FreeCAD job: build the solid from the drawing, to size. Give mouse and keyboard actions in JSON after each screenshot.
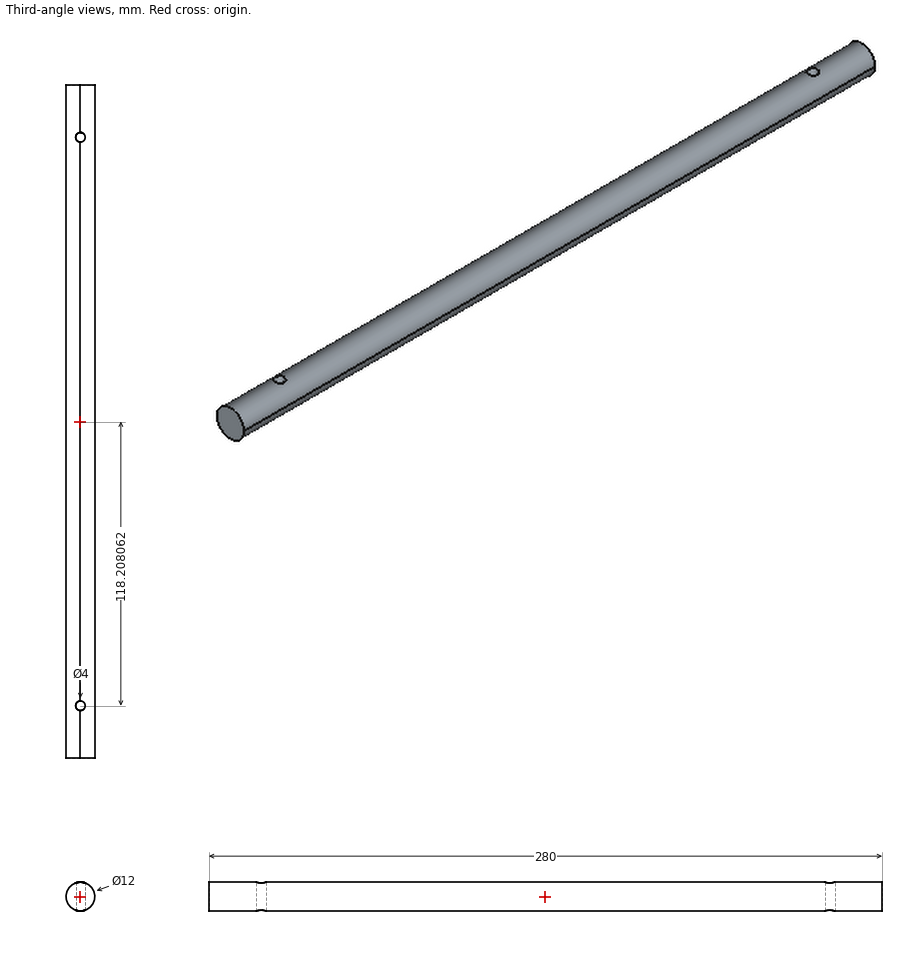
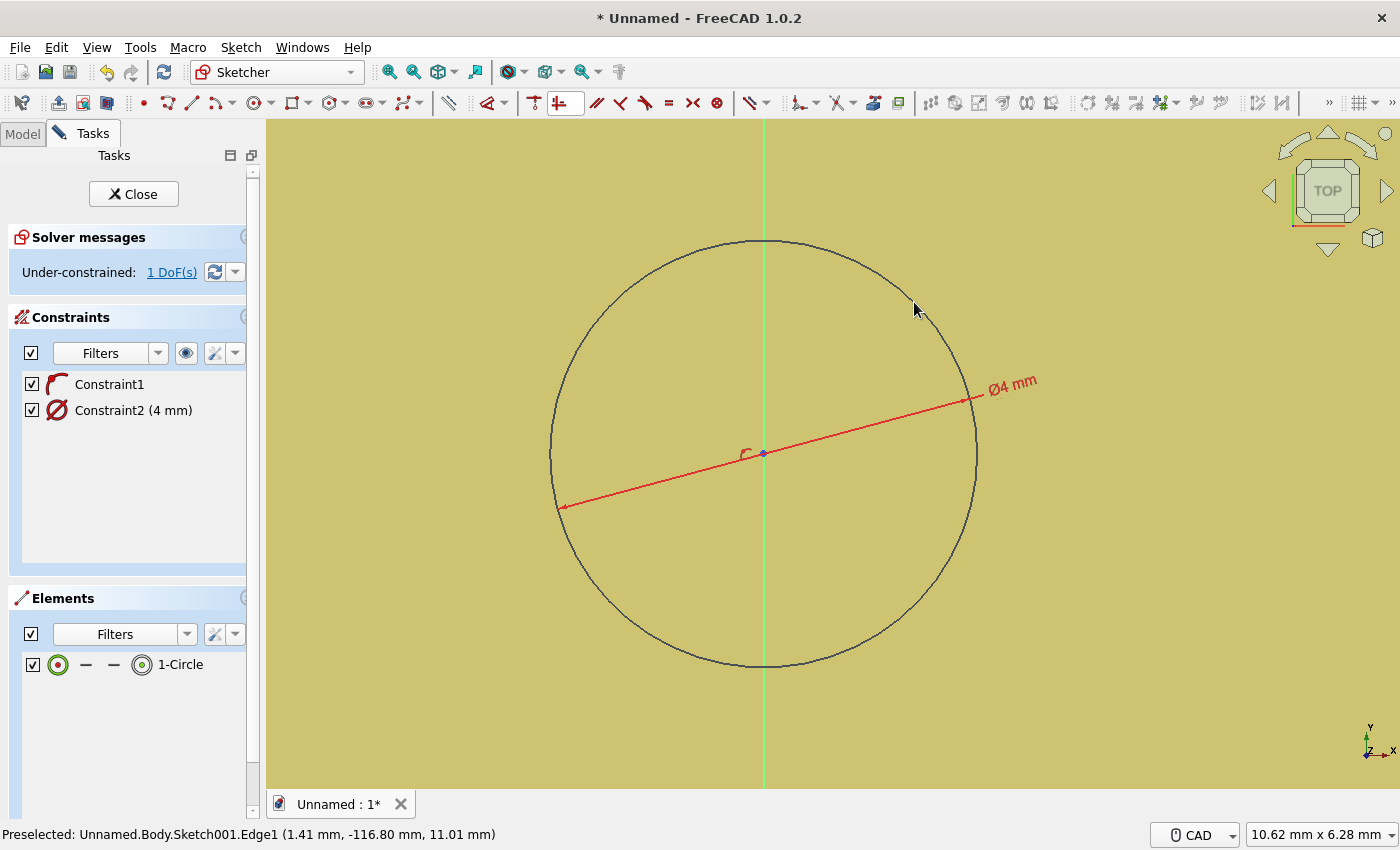
{"action": "left_click", "coordinate": [764, 454]}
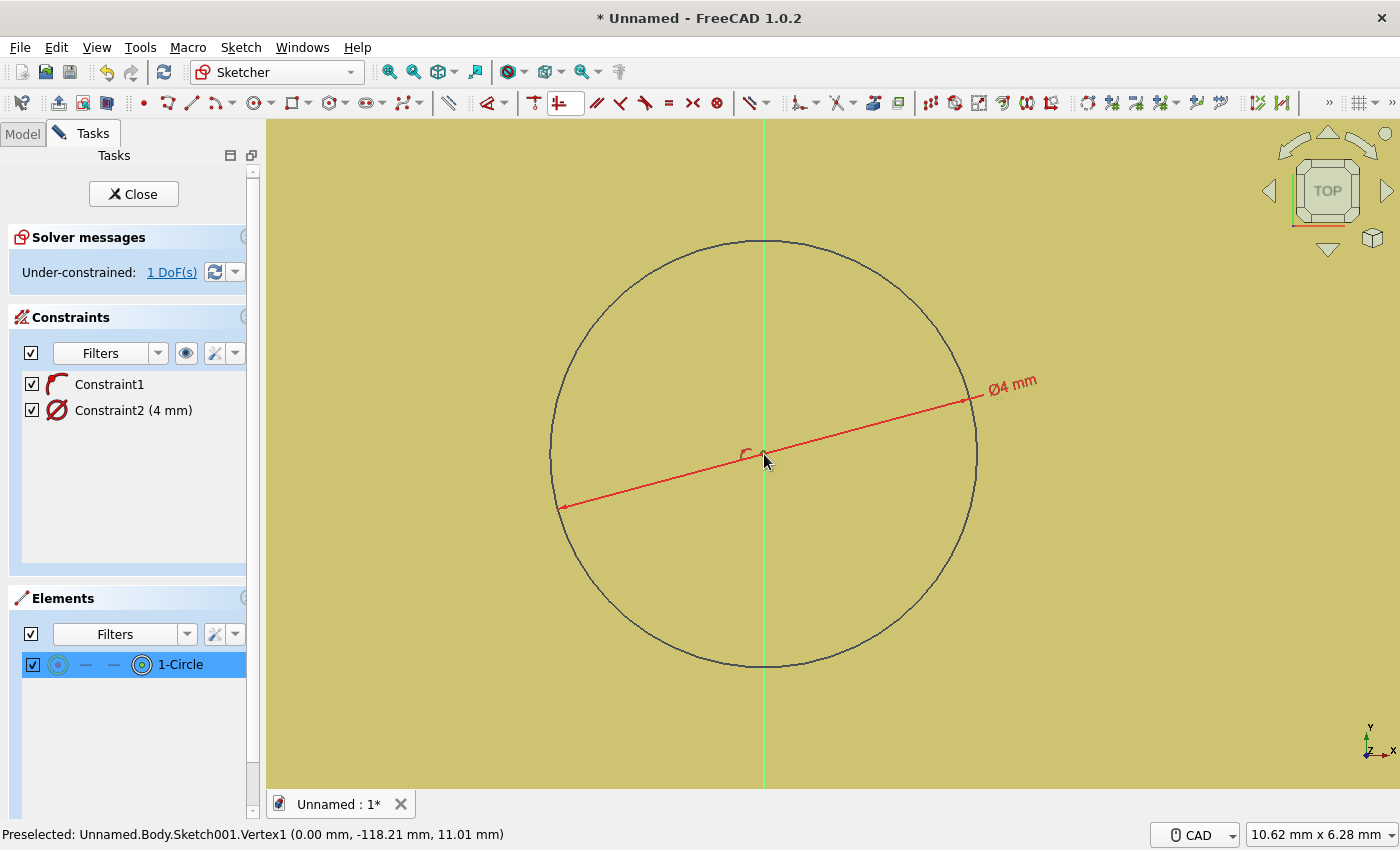
{"action": "left_click", "coordinate": [506, 104]}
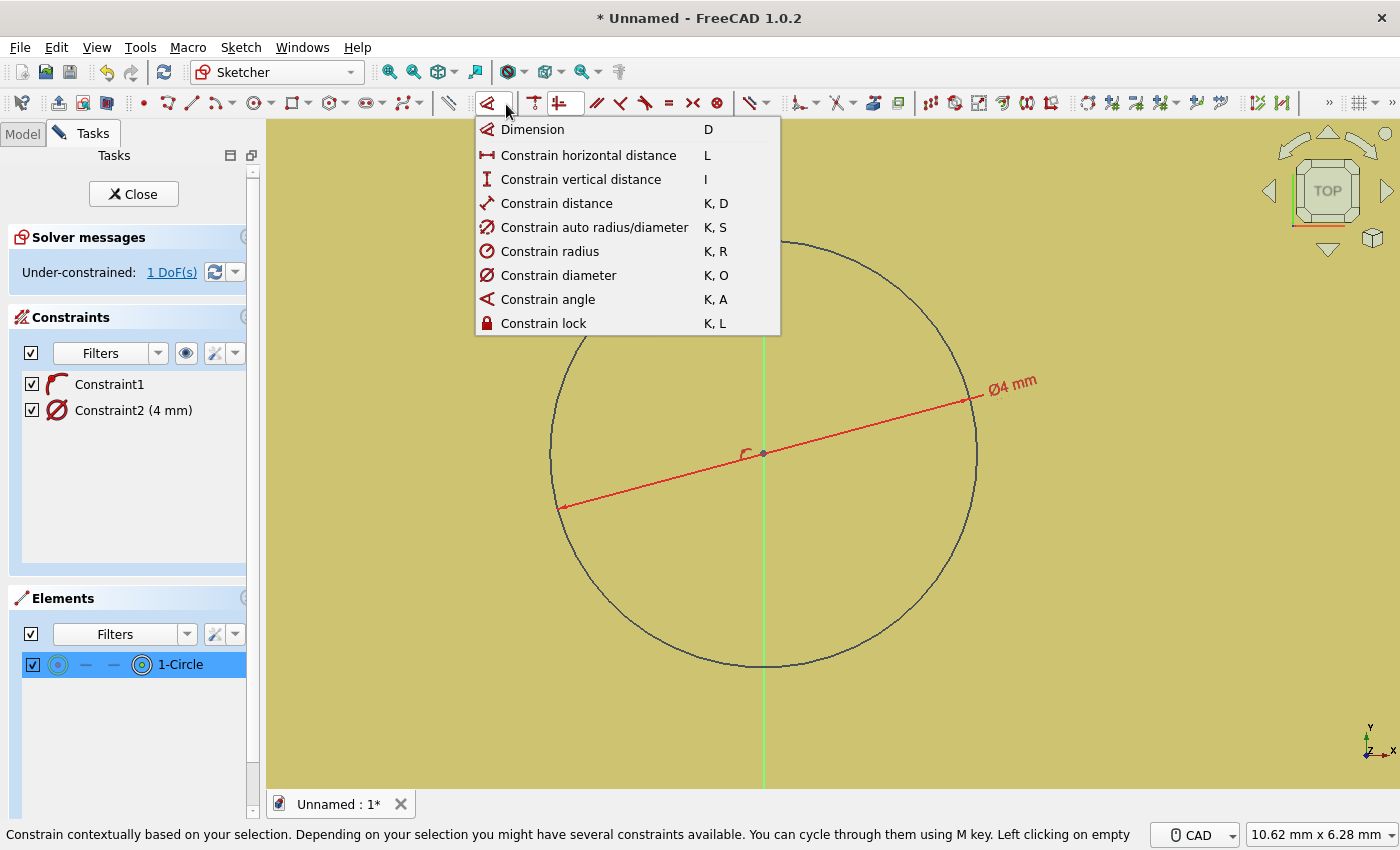
{"action": "left_click", "coordinate": [628, 179]}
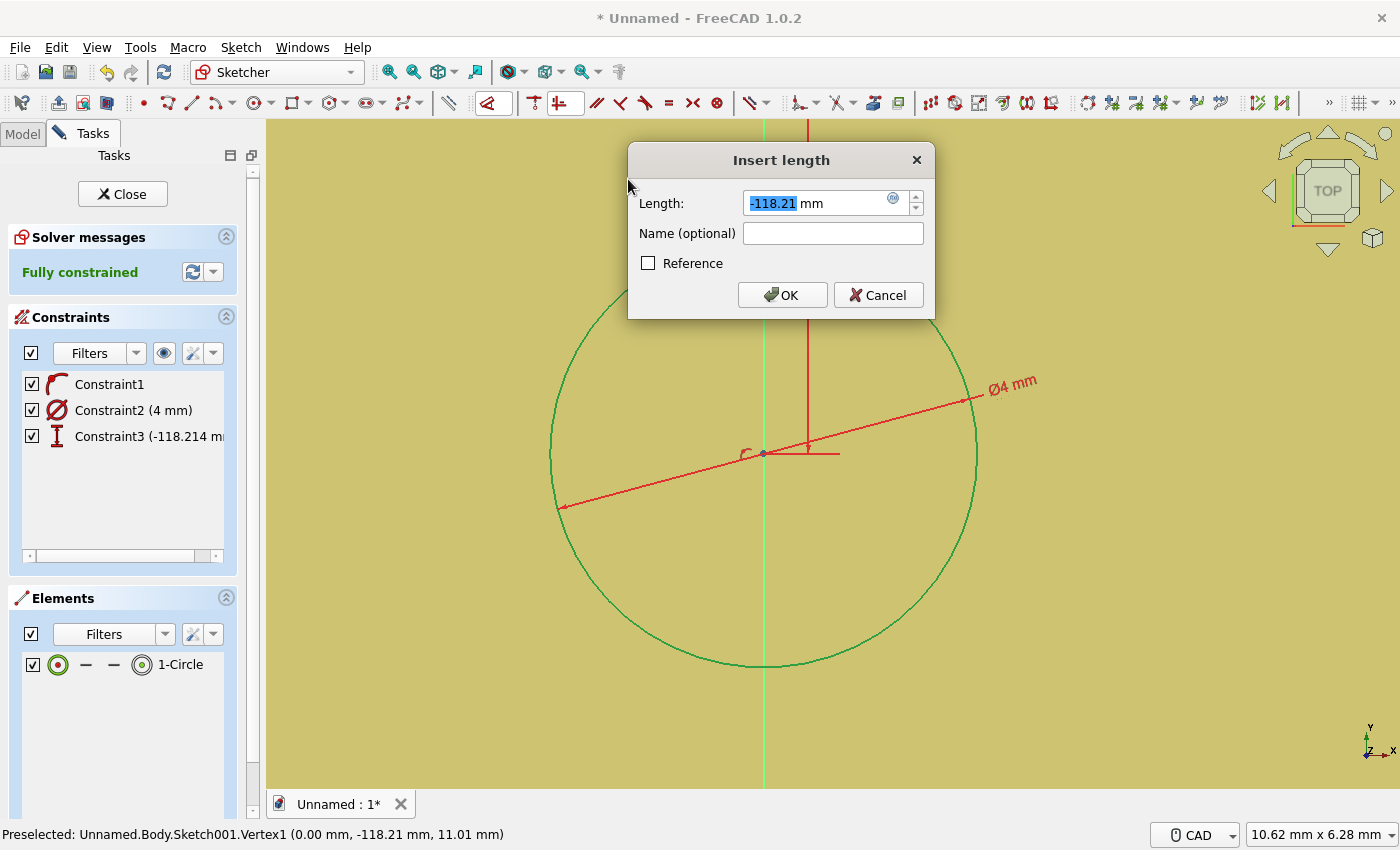
{"action": "type", "text": "-118.208062"}
{"action": "key", "text": "Return"}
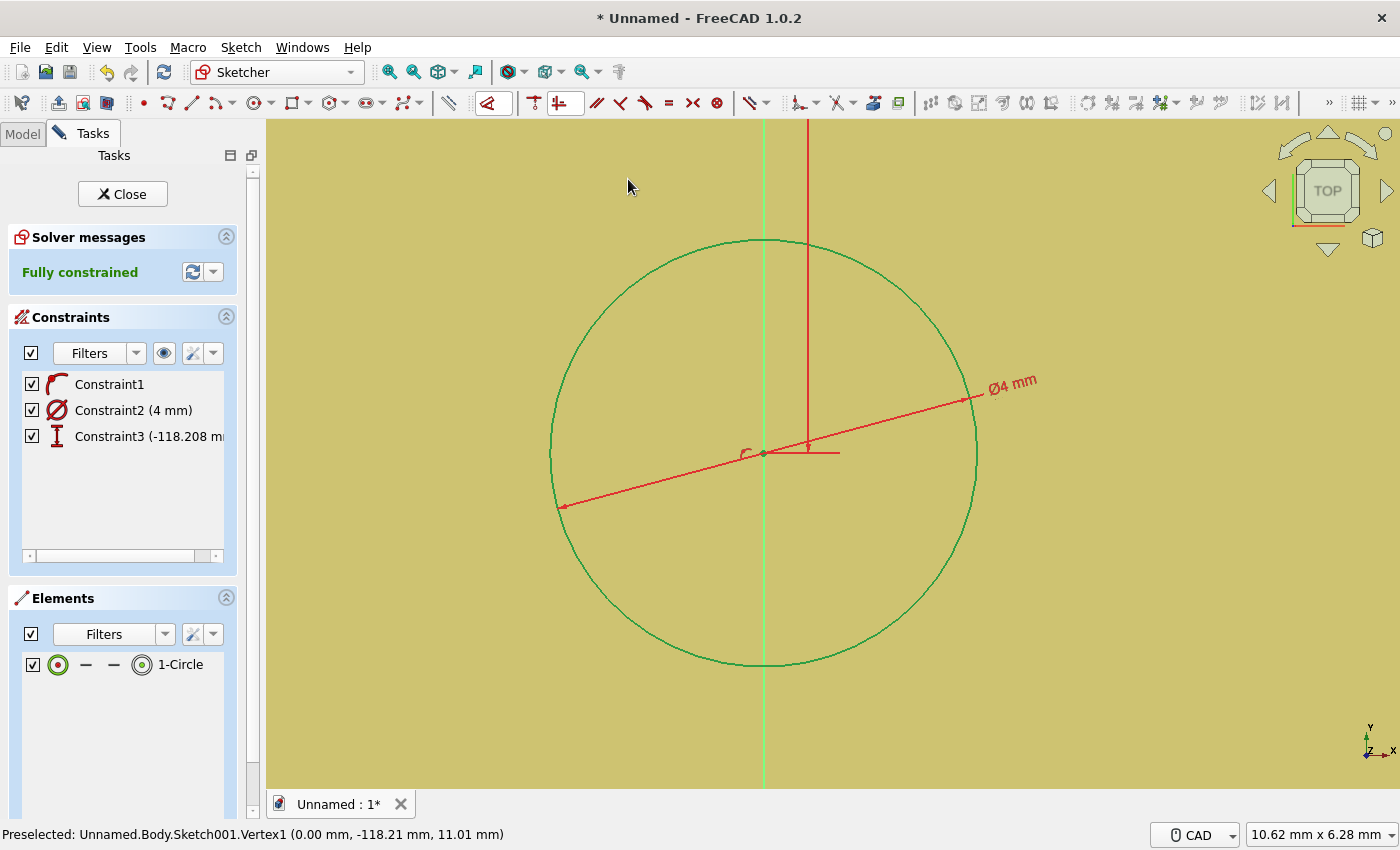
{"action": "left_click", "coordinate": [123, 194]}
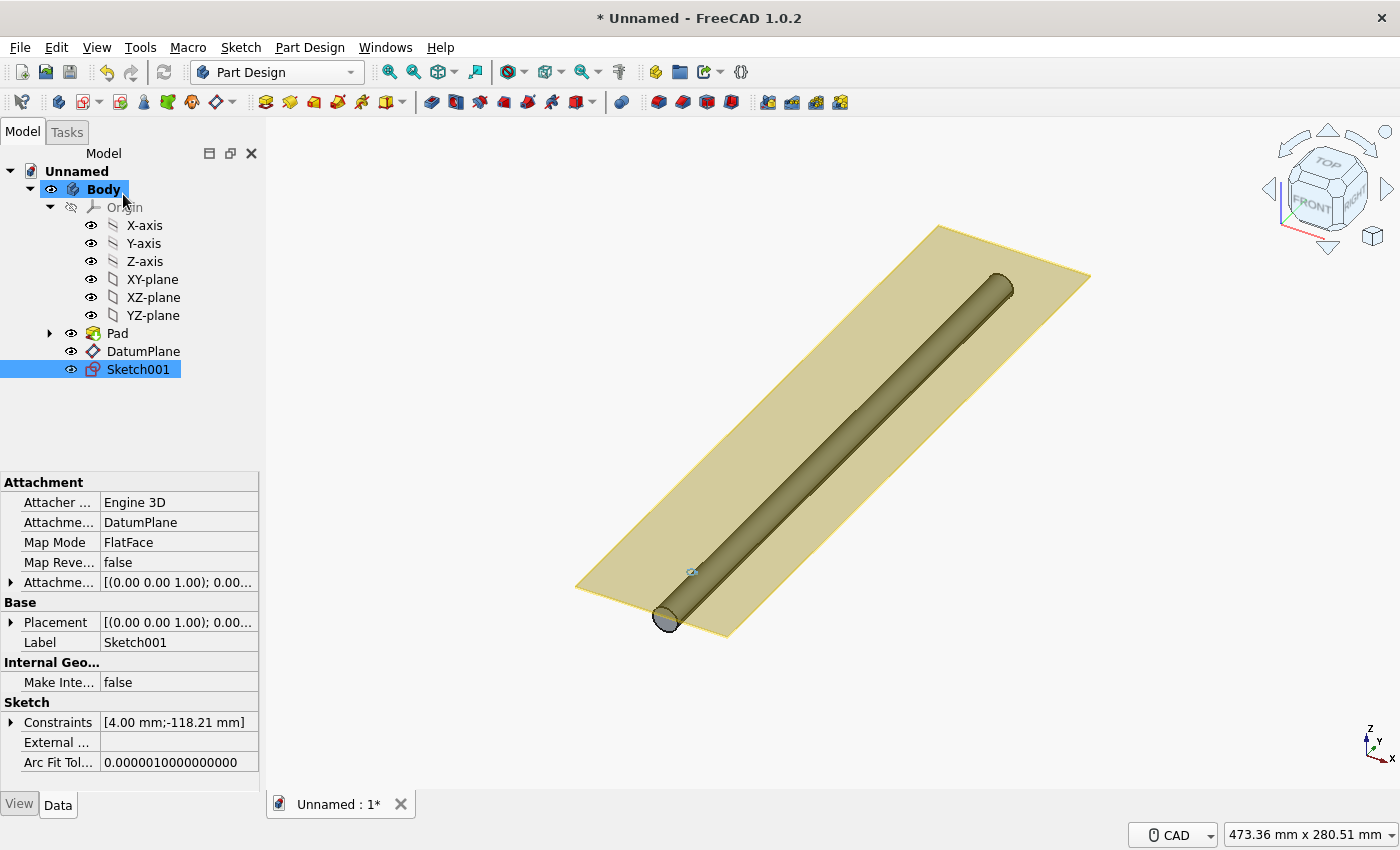
{"action": "left_click", "coordinate": [432, 102]}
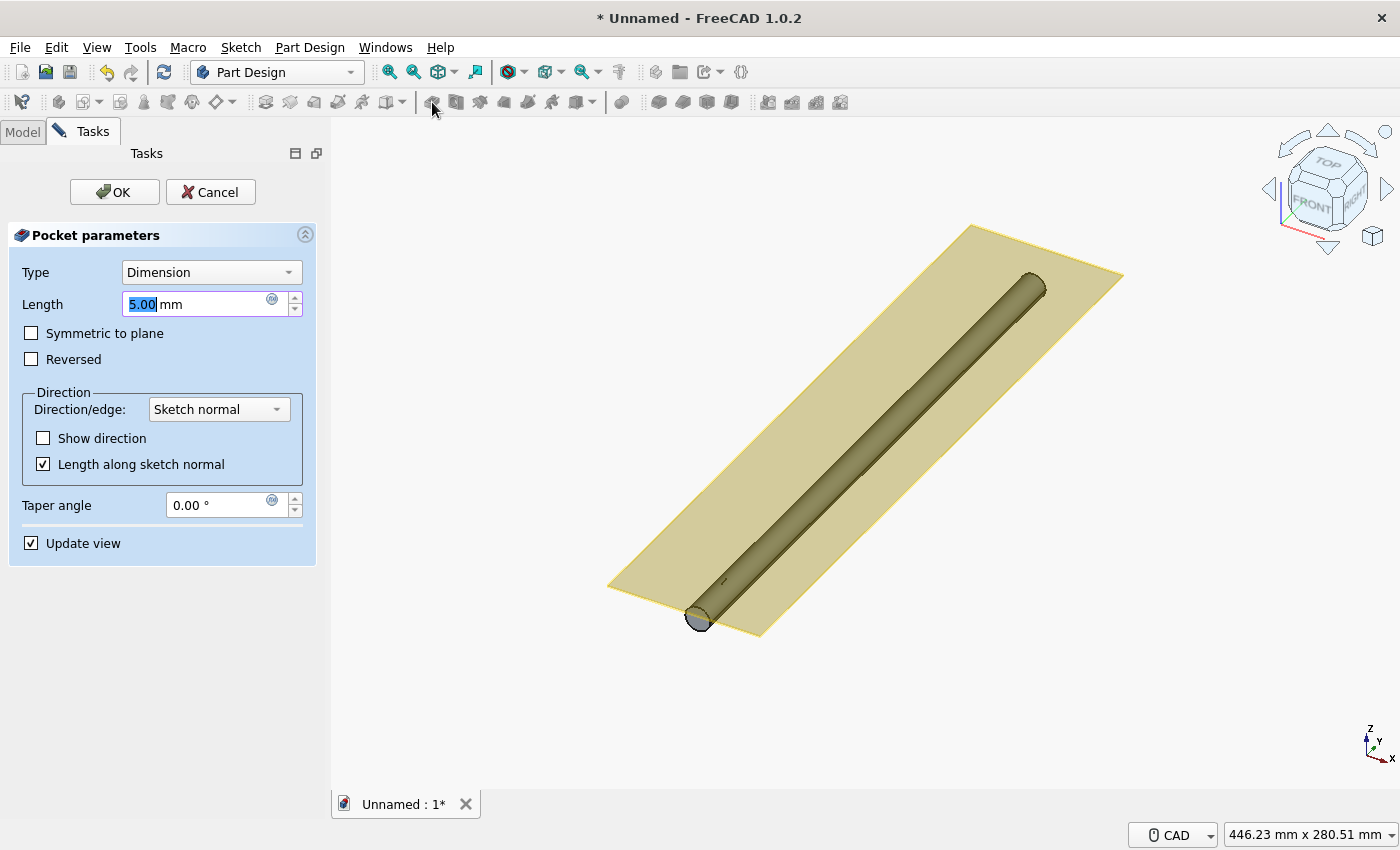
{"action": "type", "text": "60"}
{"action": "key", "text": "Tab"}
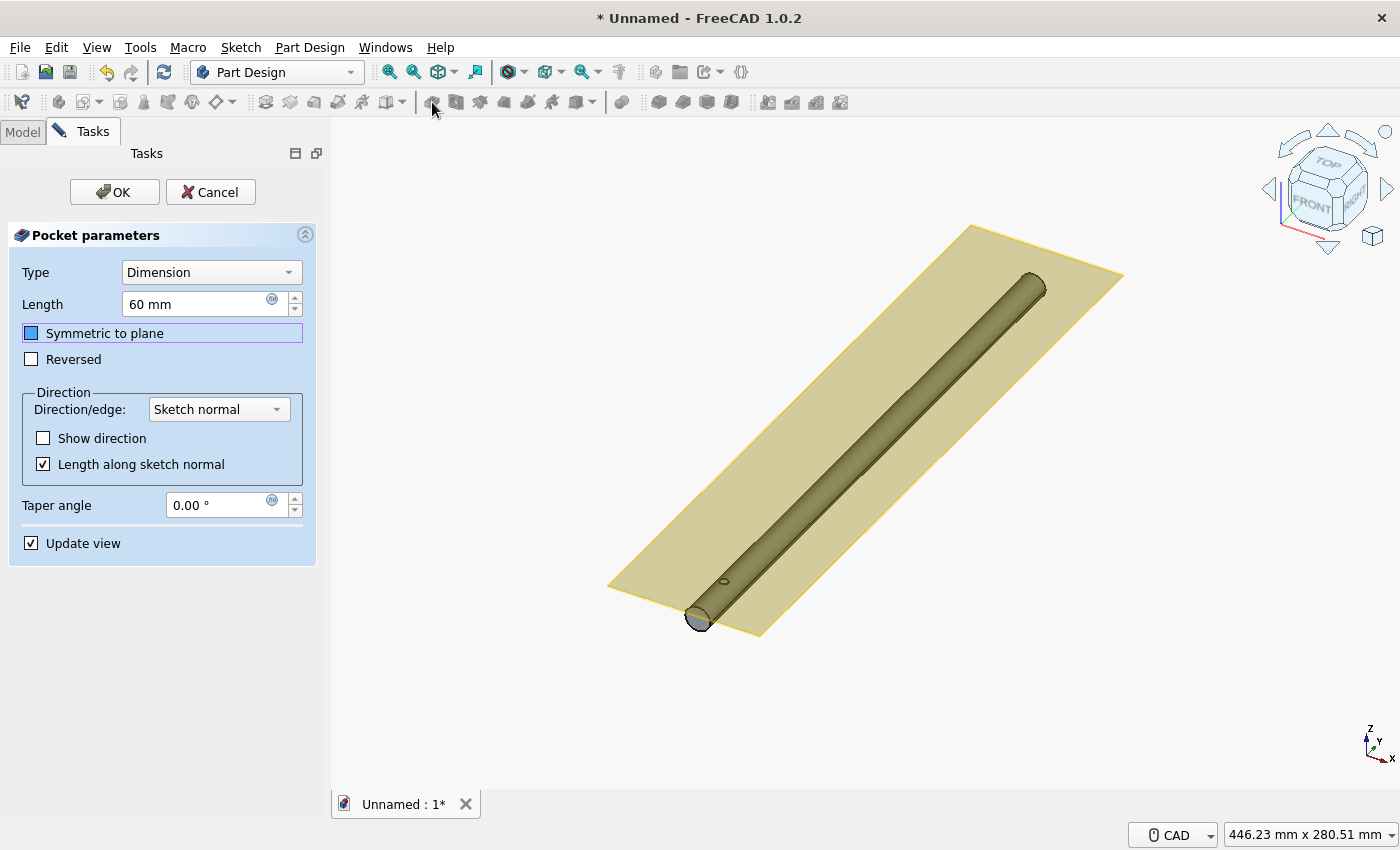
{"action": "left_click", "coordinate": [115, 192]}